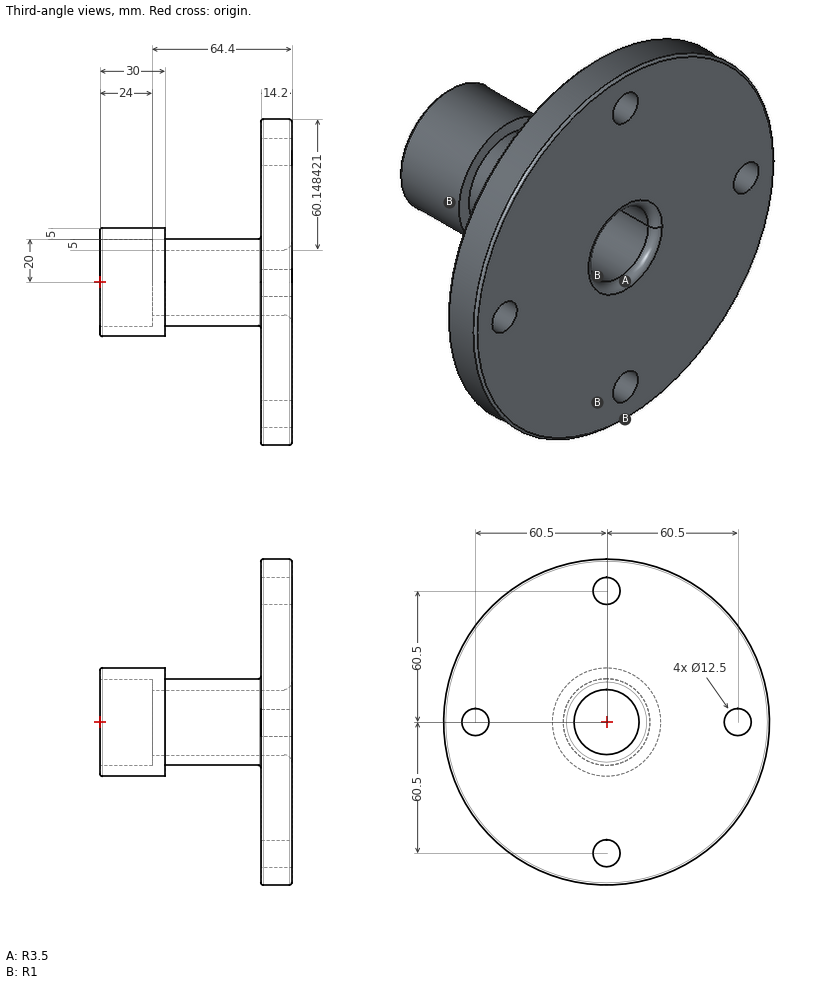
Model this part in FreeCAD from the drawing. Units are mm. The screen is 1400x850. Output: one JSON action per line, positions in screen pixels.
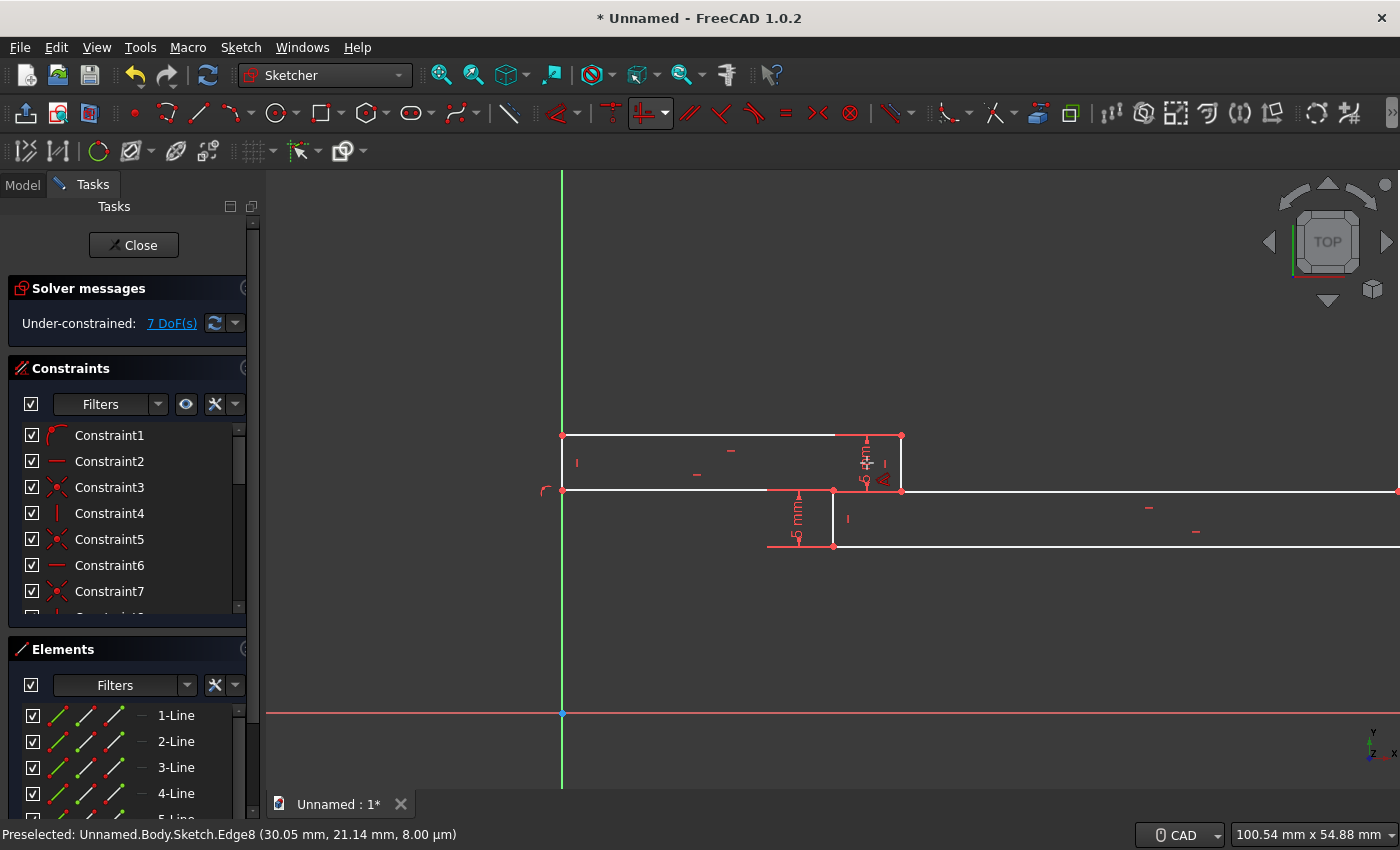
{"action": "left_click", "coordinate": [562, 452]}
{"action": "left_click", "coordinate": [528, 463]}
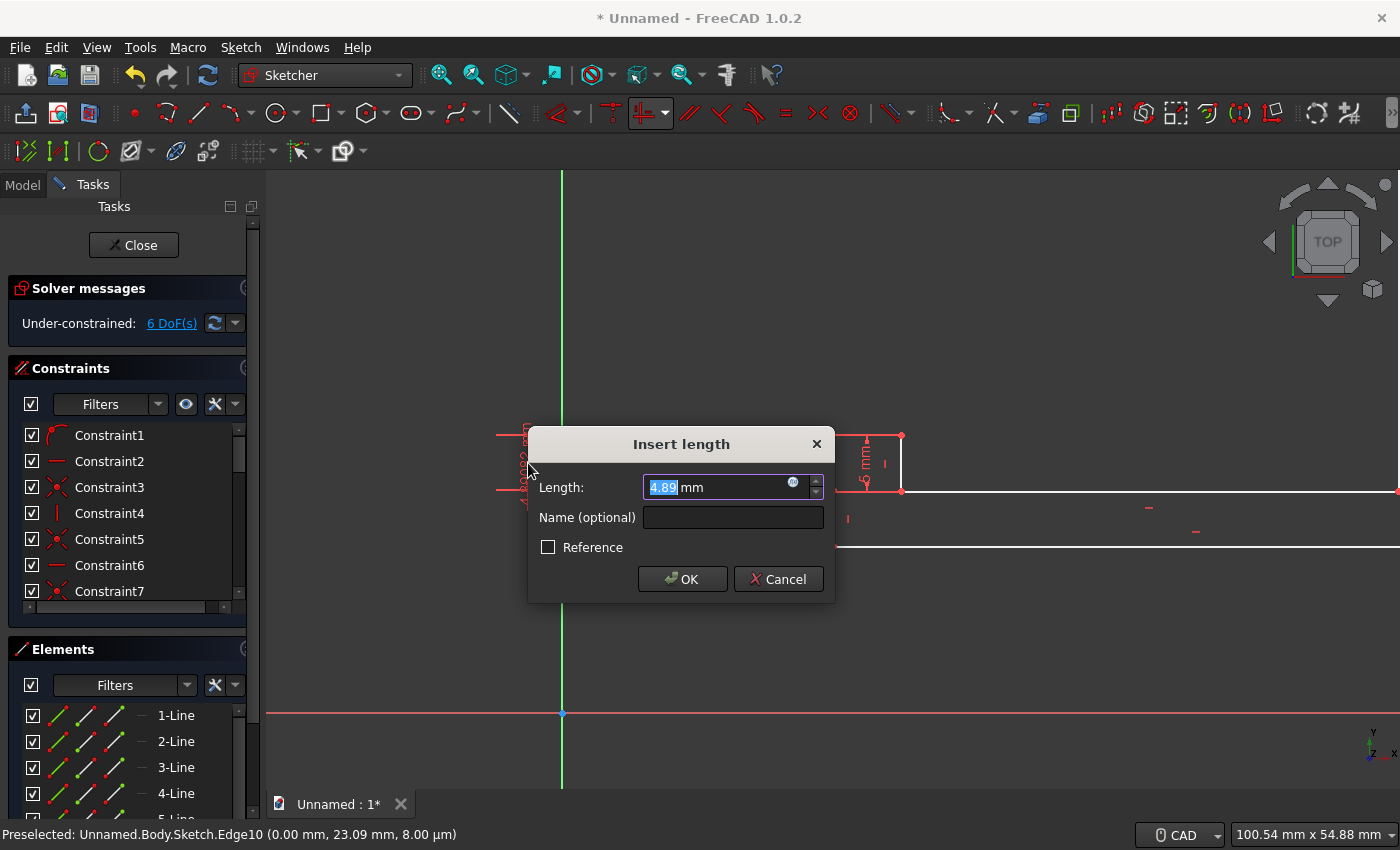
{"action": "type", "text": "5"}
{"action": "key", "text": "Return"}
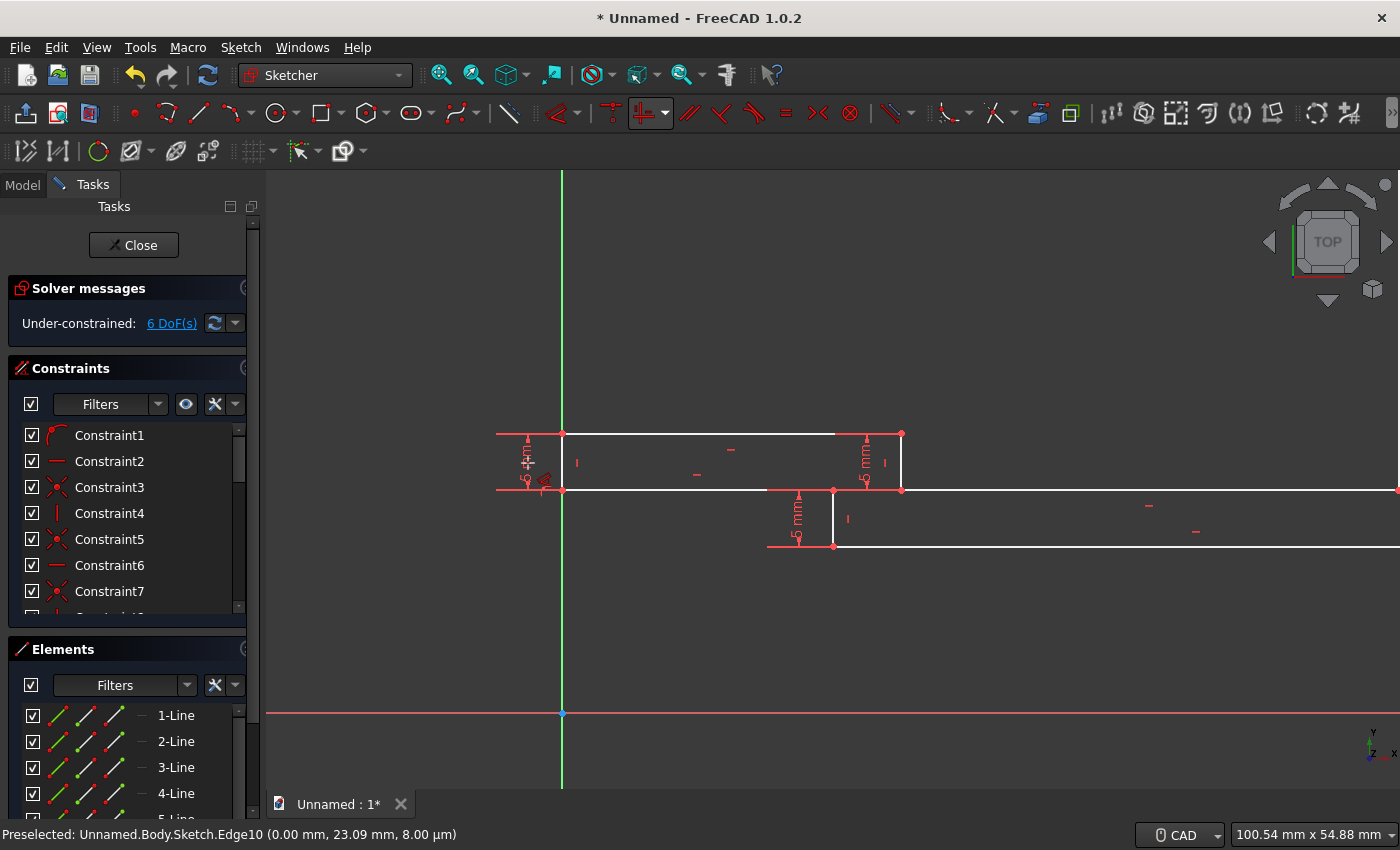
{"action": "left_click", "coordinate": [644, 490]}
{"action": "left_click", "coordinate": [698, 524]}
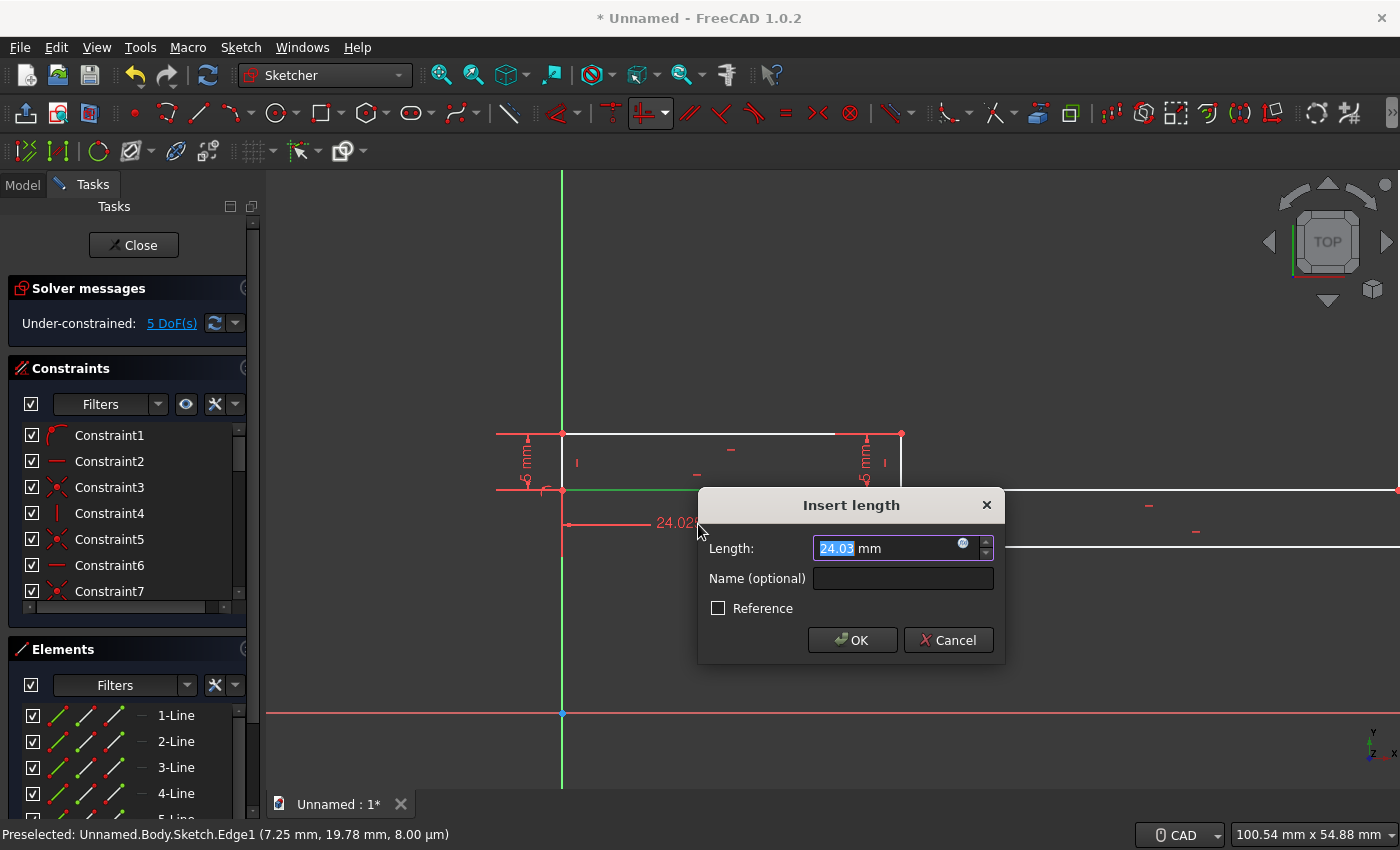
{"action": "type", "text": "24"}
{"action": "key", "text": "Return"}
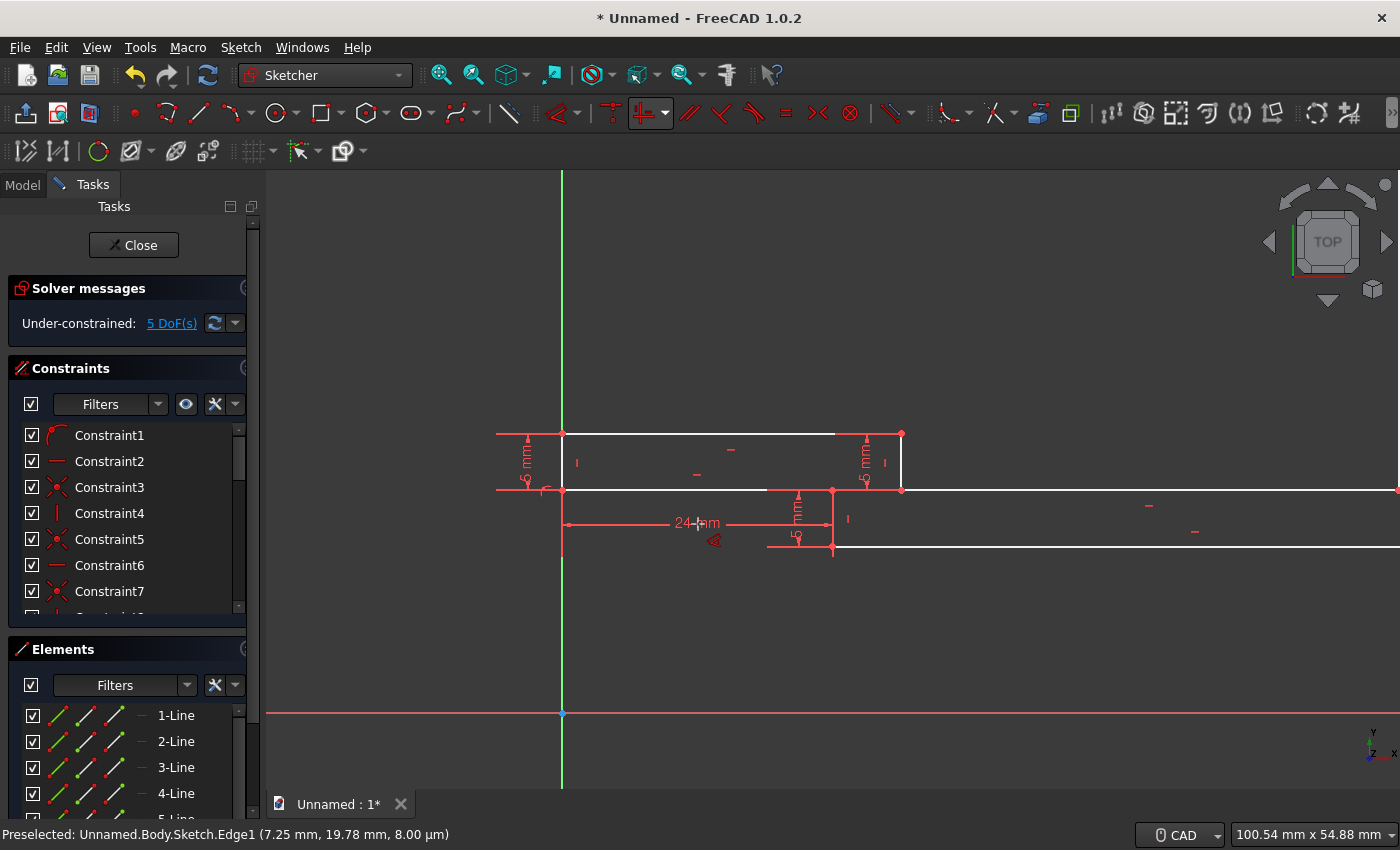
{"action": "left_click", "coordinate": [799, 434]}
{"action": "left_click", "coordinate": [732, 468]}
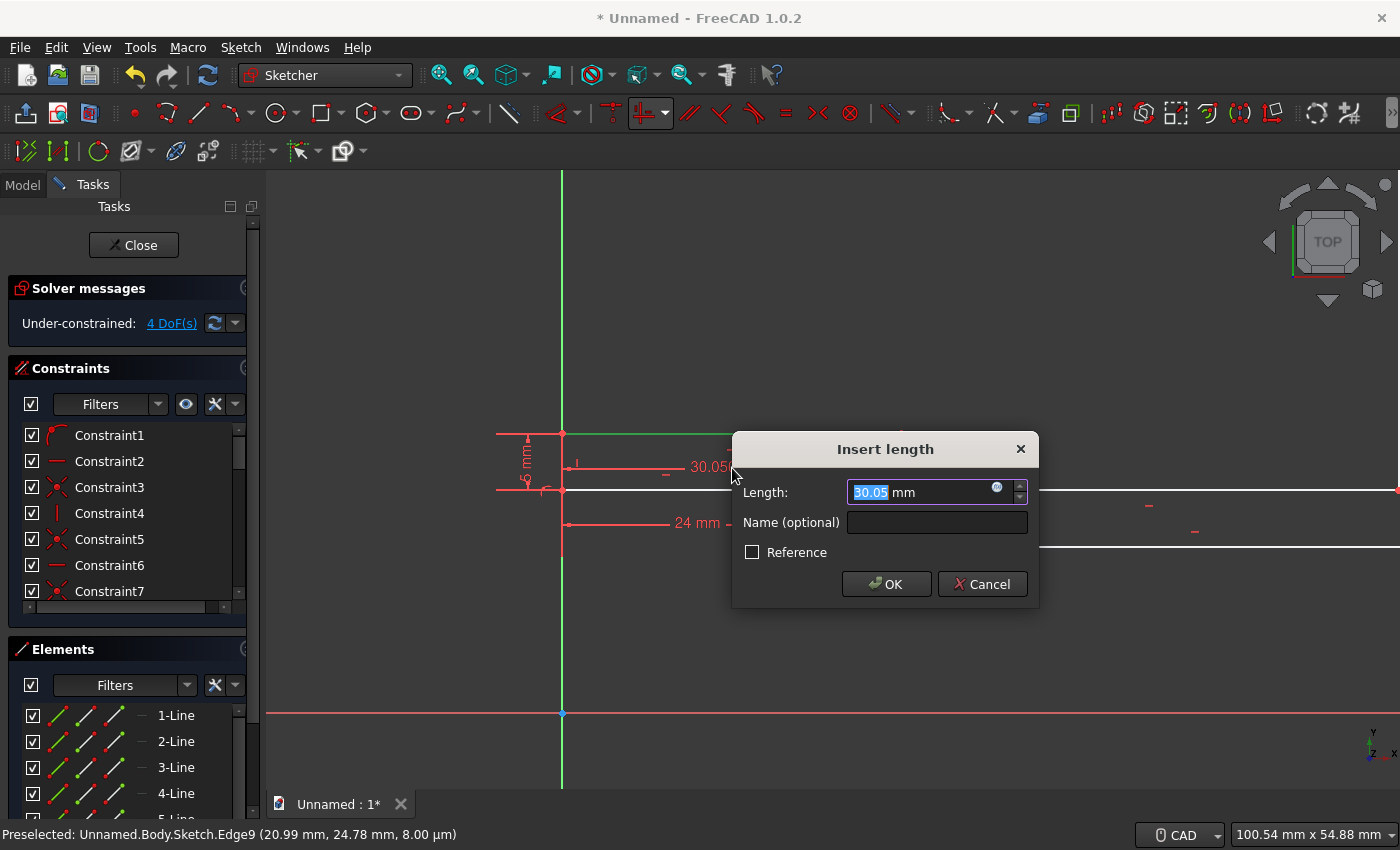
{"action": "type", "text": "30"}
{"action": "key", "text": "Return"}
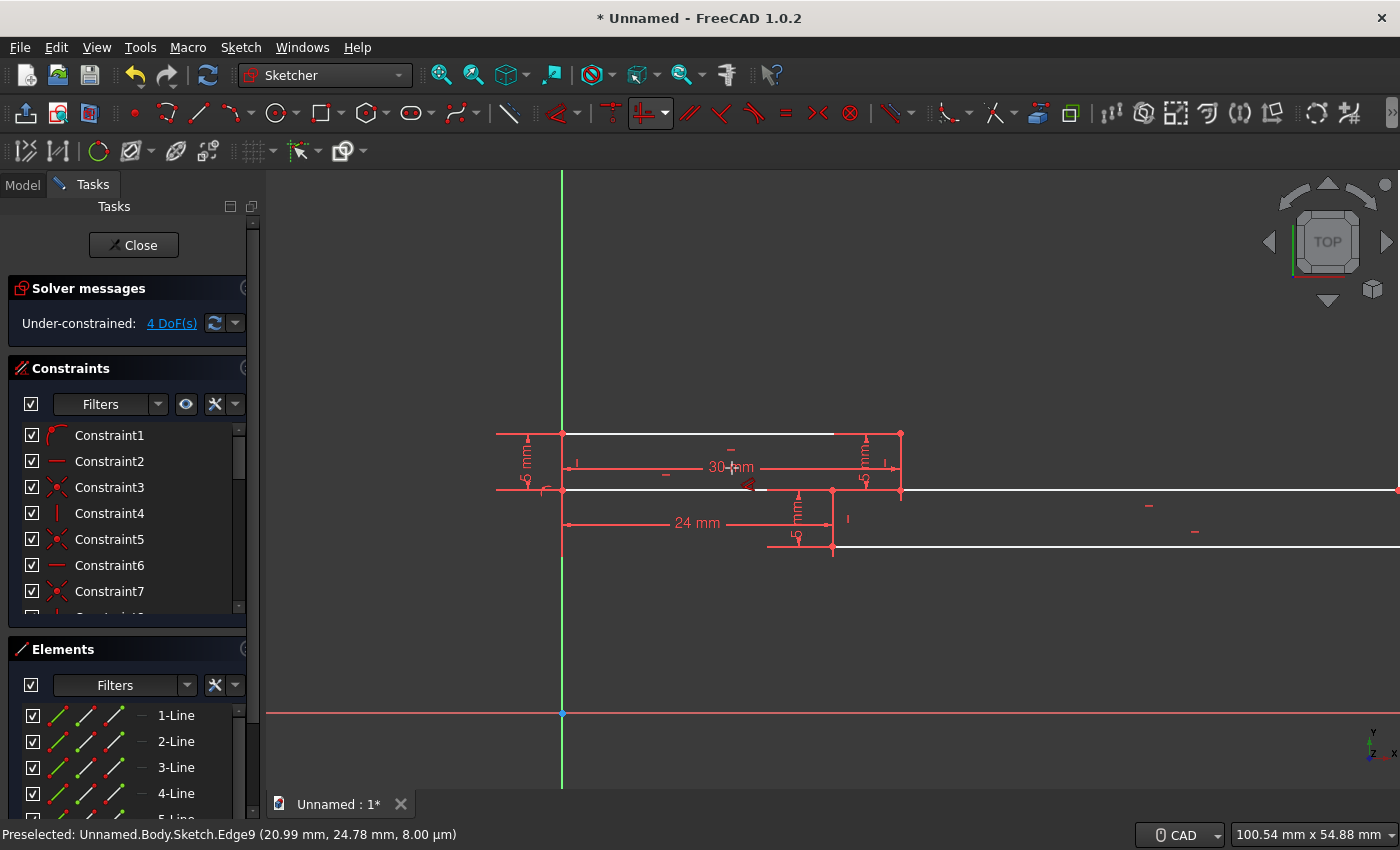
{"action": "left_click", "coordinate": [562, 490]}
{"action": "left_click", "coordinate": [528, 602]}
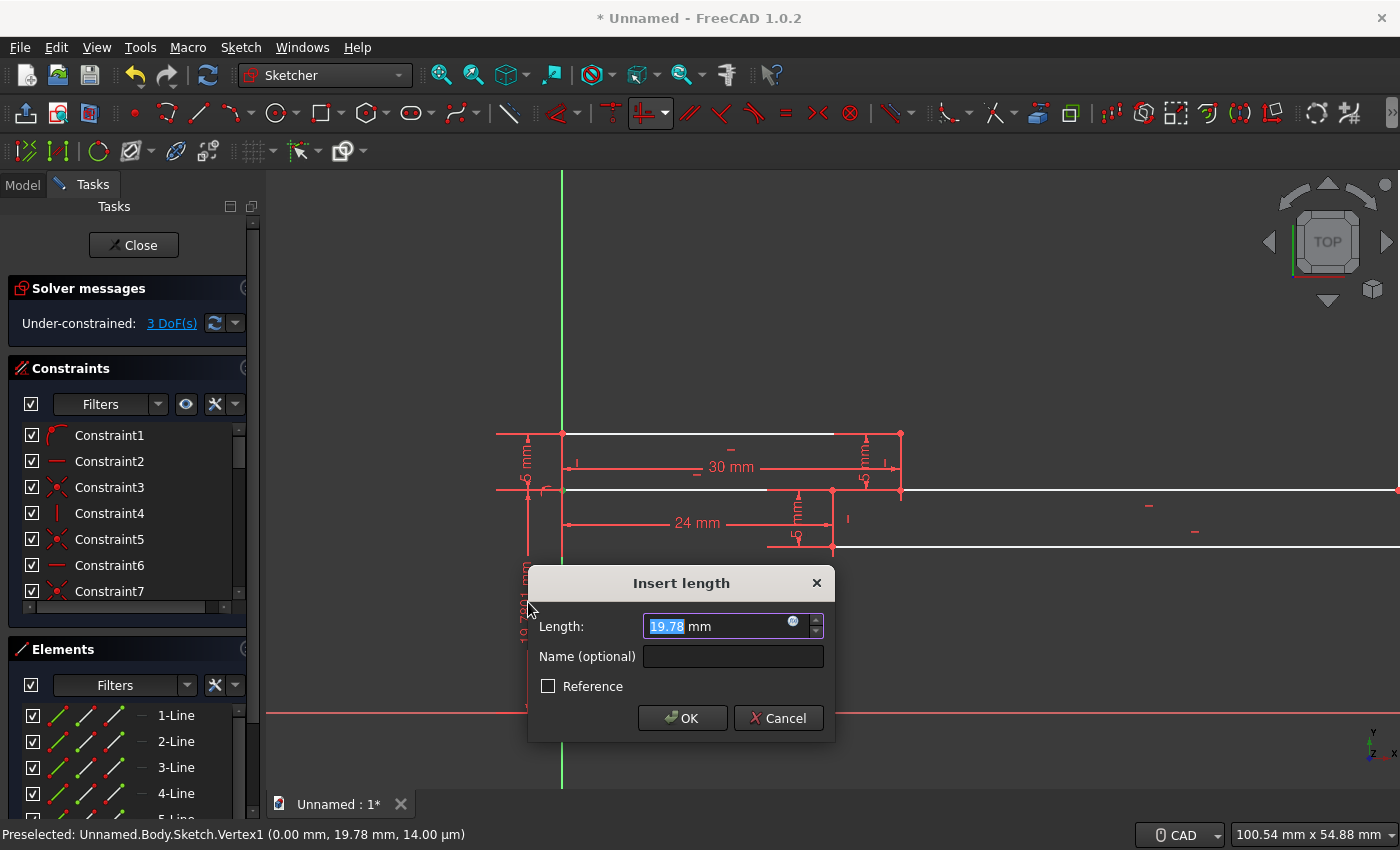
{"action": "type", "text": "20"}
{"action": "key", "text": "Return"}